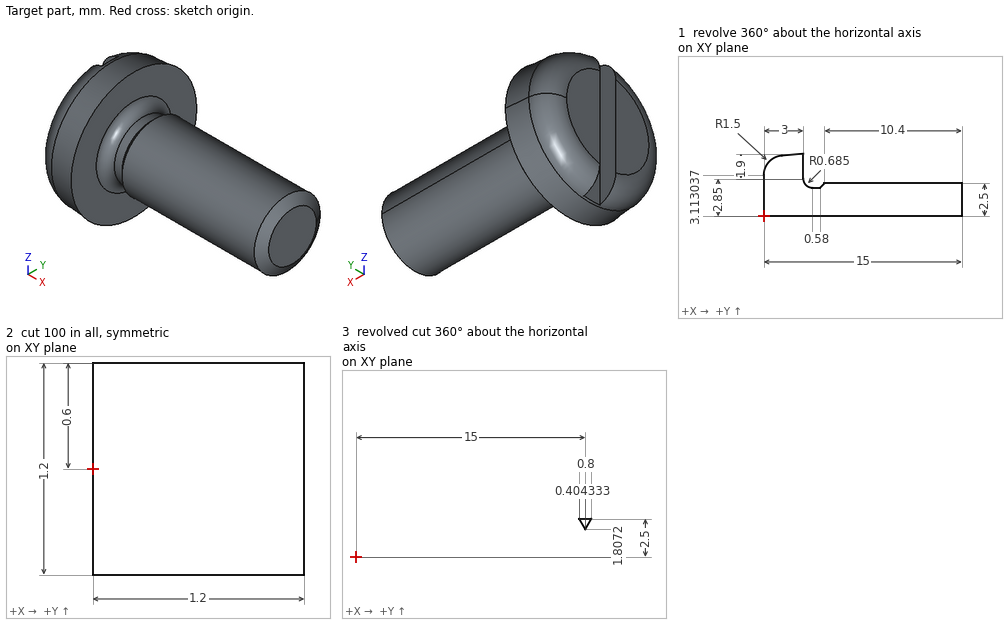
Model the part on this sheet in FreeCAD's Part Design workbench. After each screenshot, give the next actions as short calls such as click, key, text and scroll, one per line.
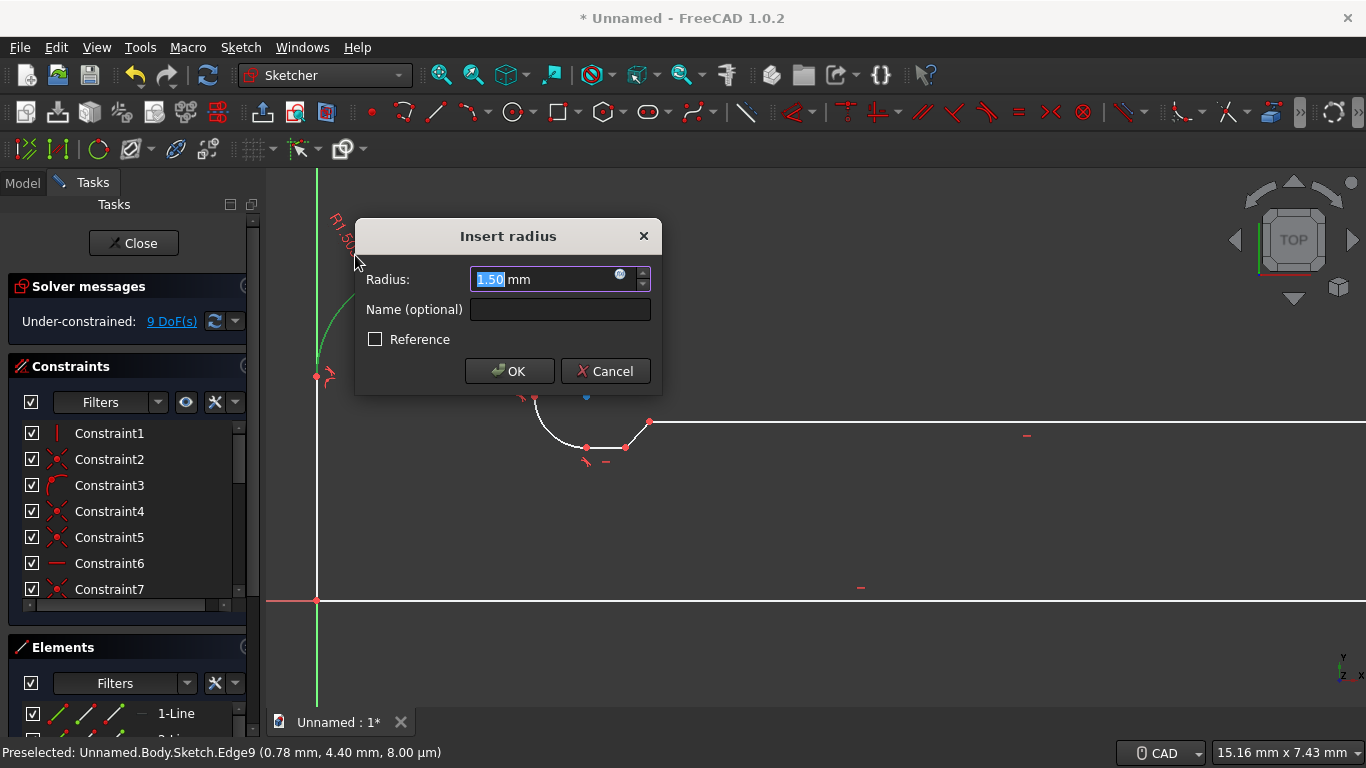
text(1.5)
key(Return)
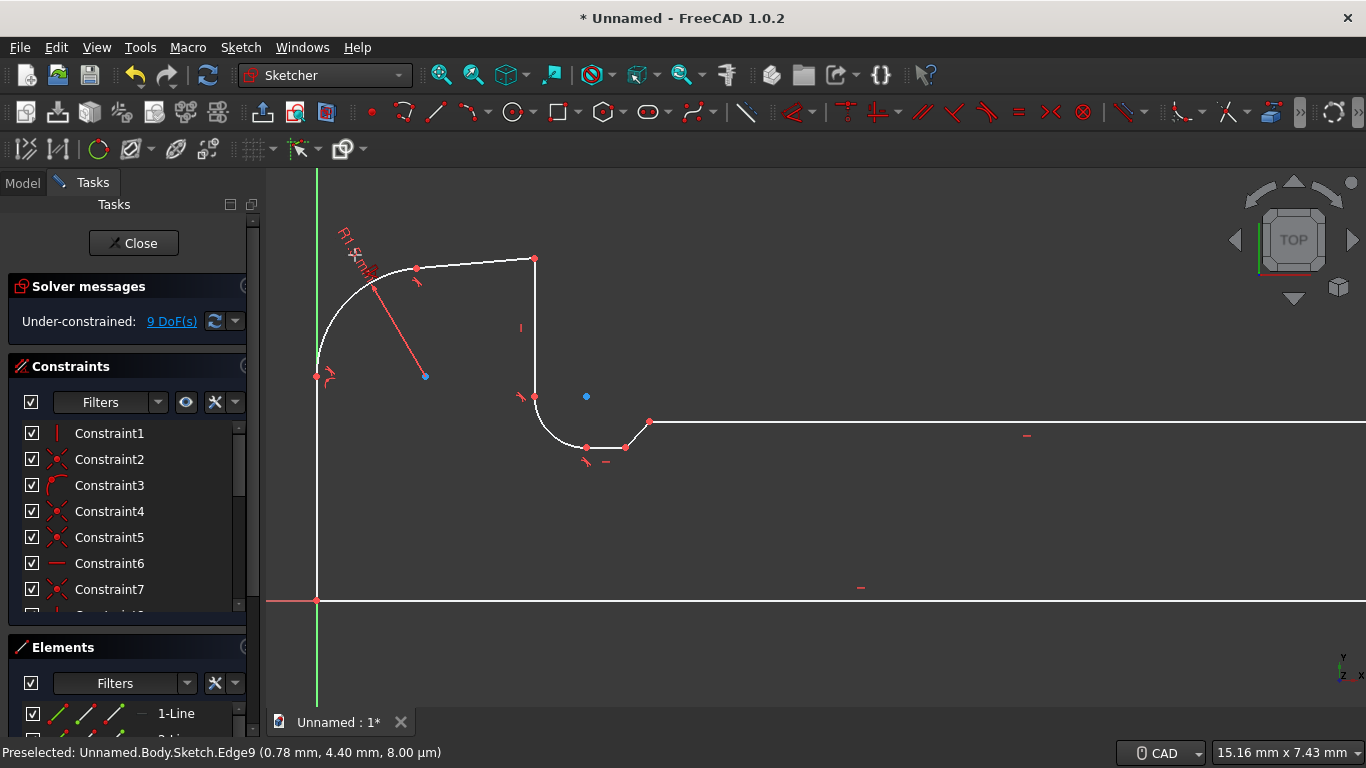
click(540, 420)
click(511, 435)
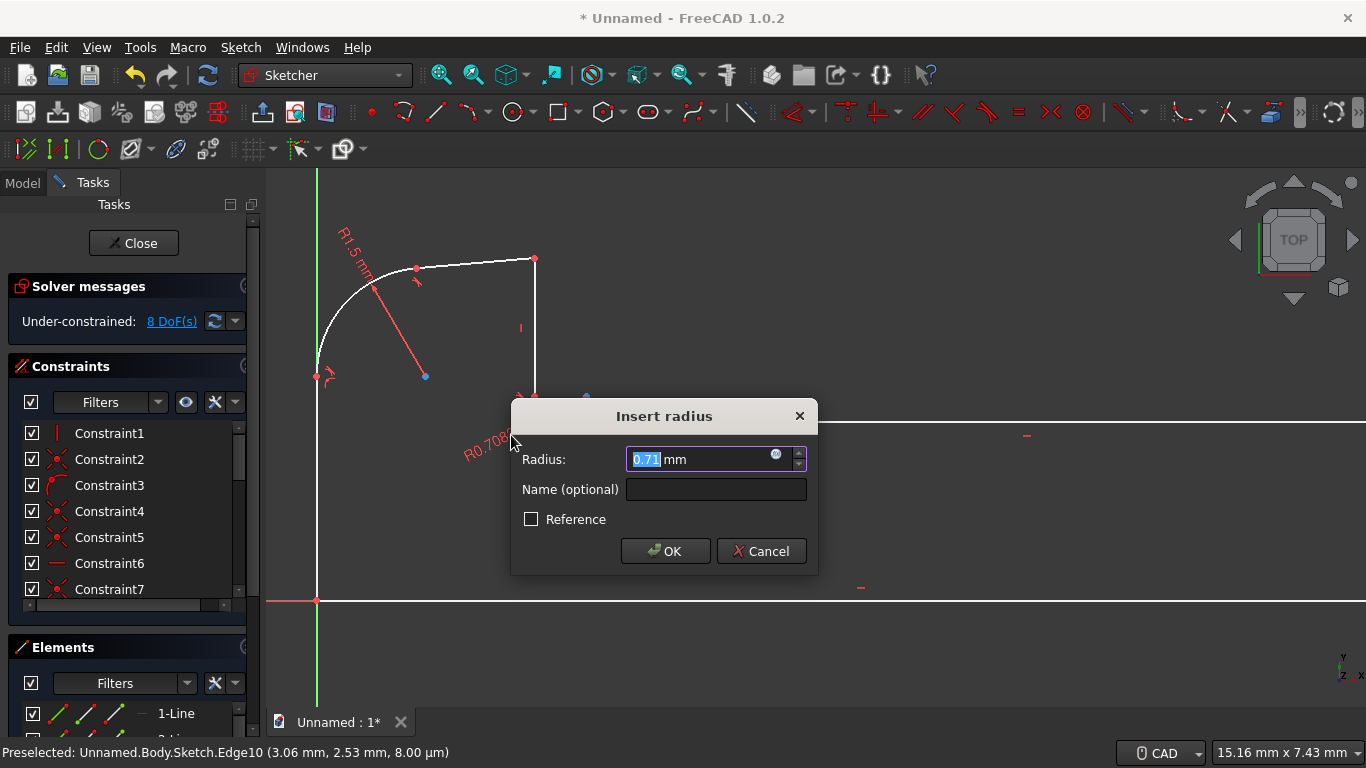
text(0.685)
key(Return)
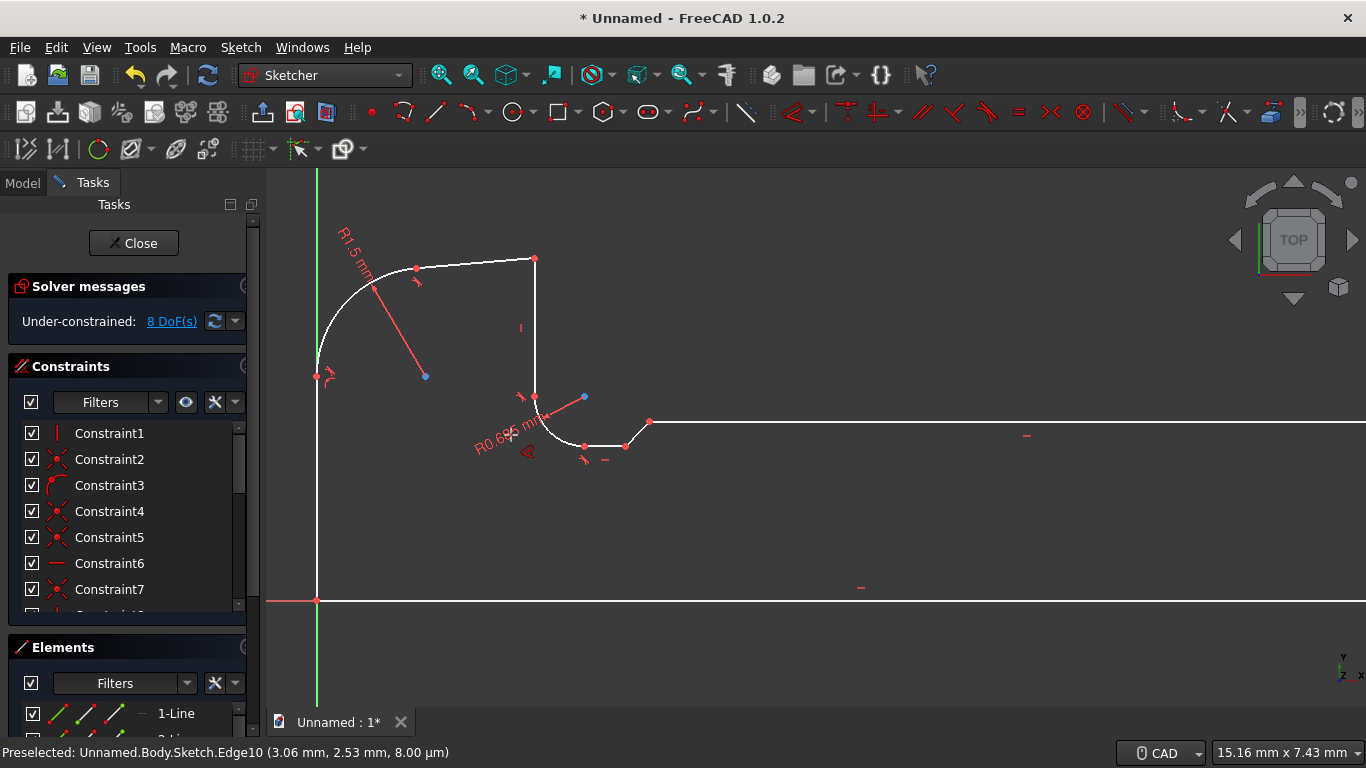
click(643, 601)
click(759, 635)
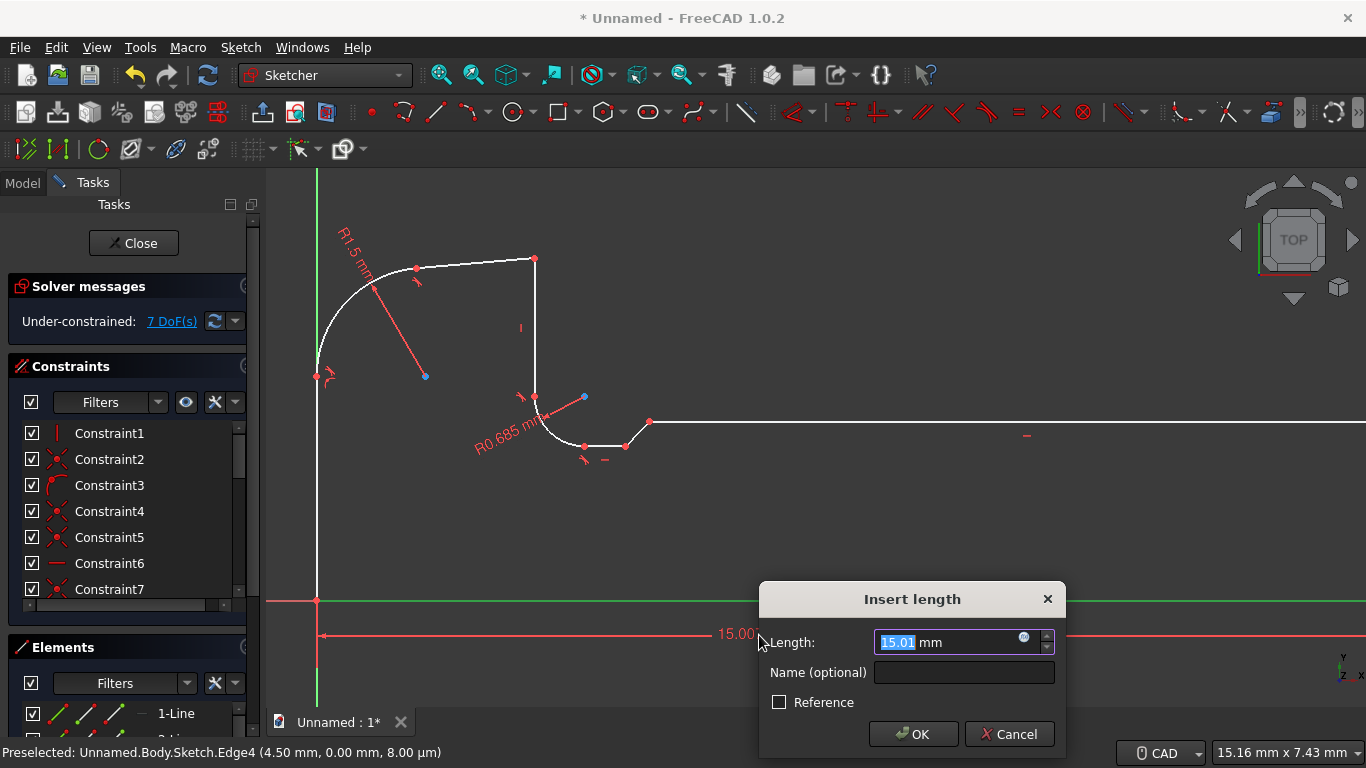
text(15)
key(Return)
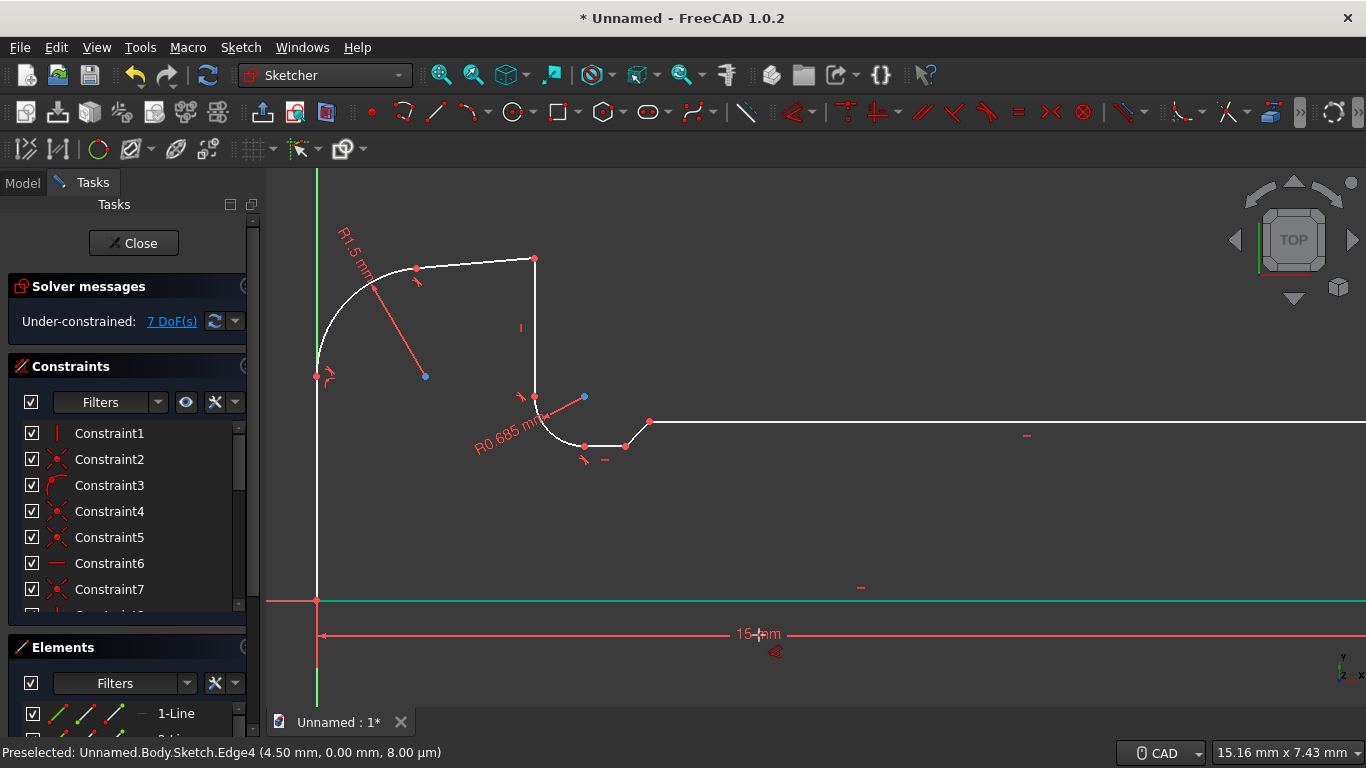
click(535, 396)
click(426, 635)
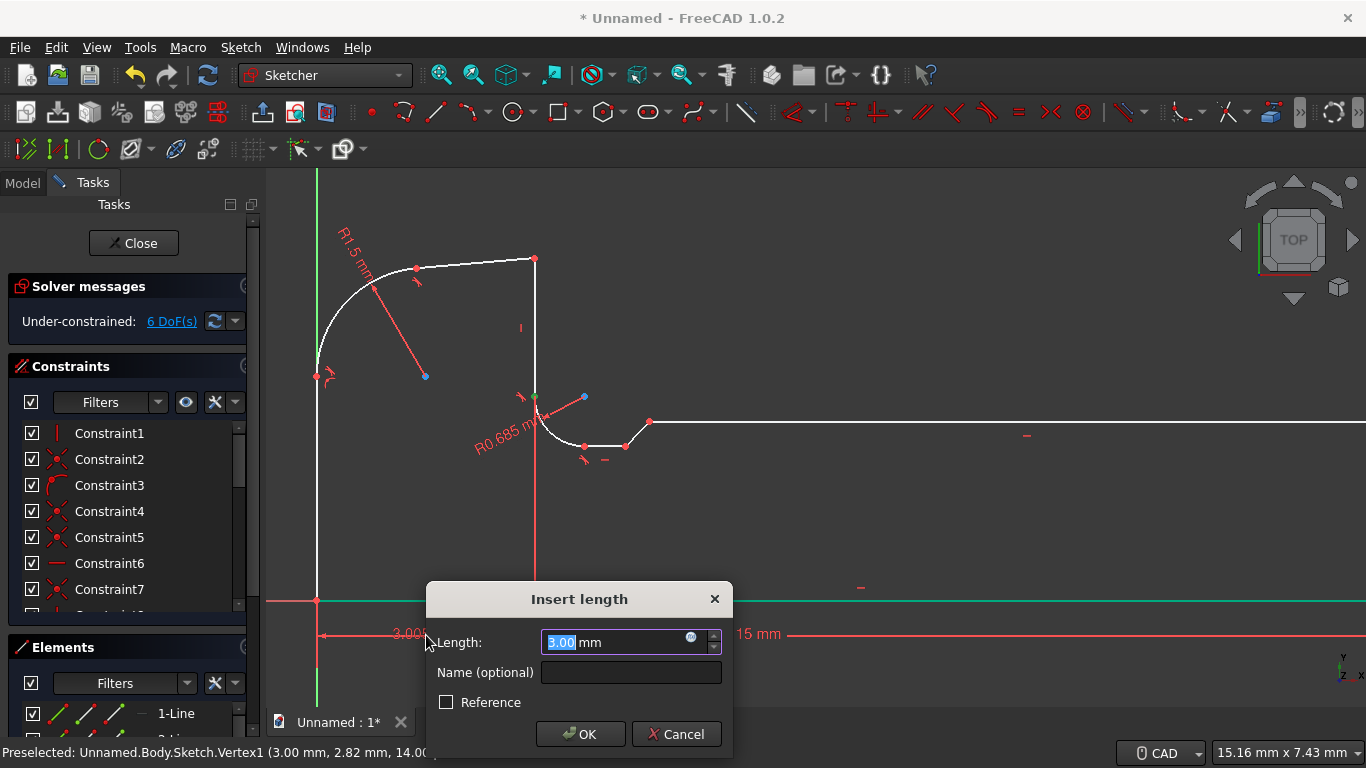
text(3)
key(Return)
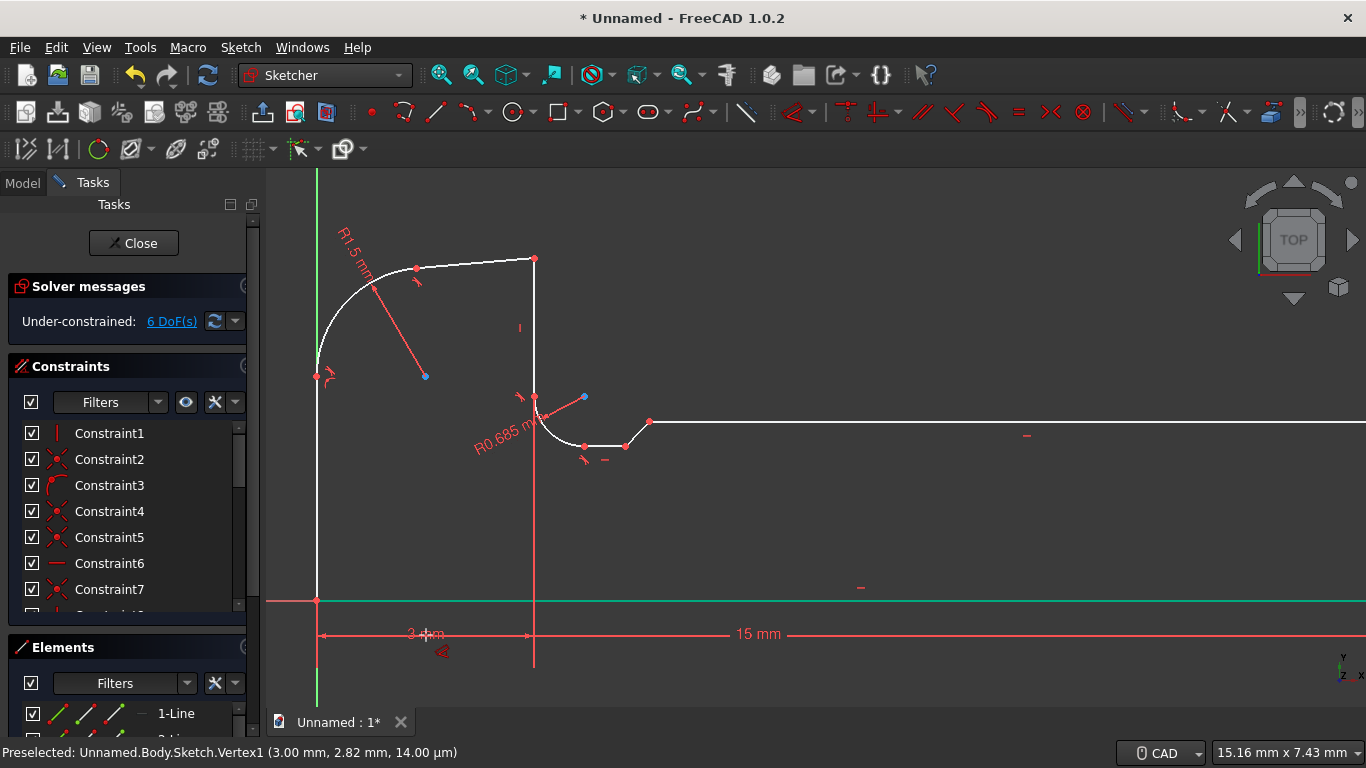
click(534, 355)
click(500, 327)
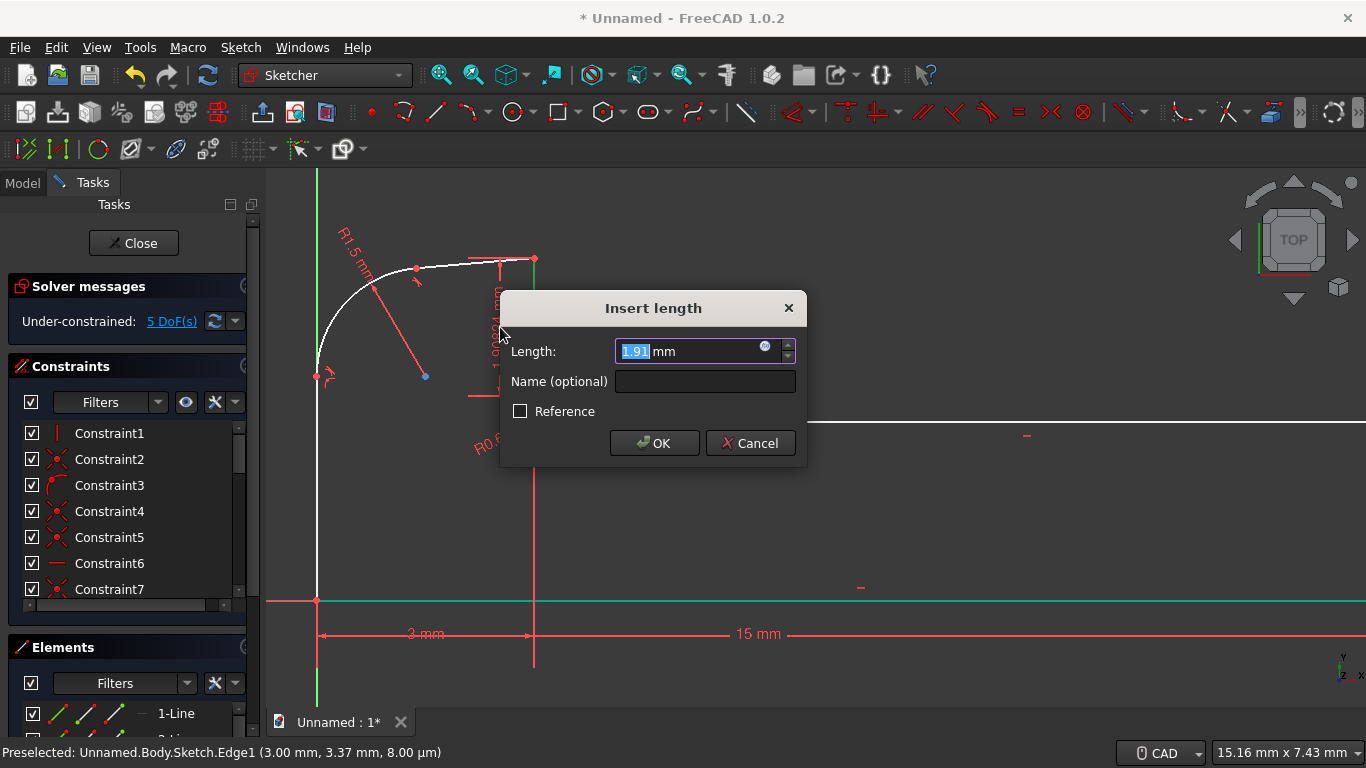
text(1.9)
key(Return)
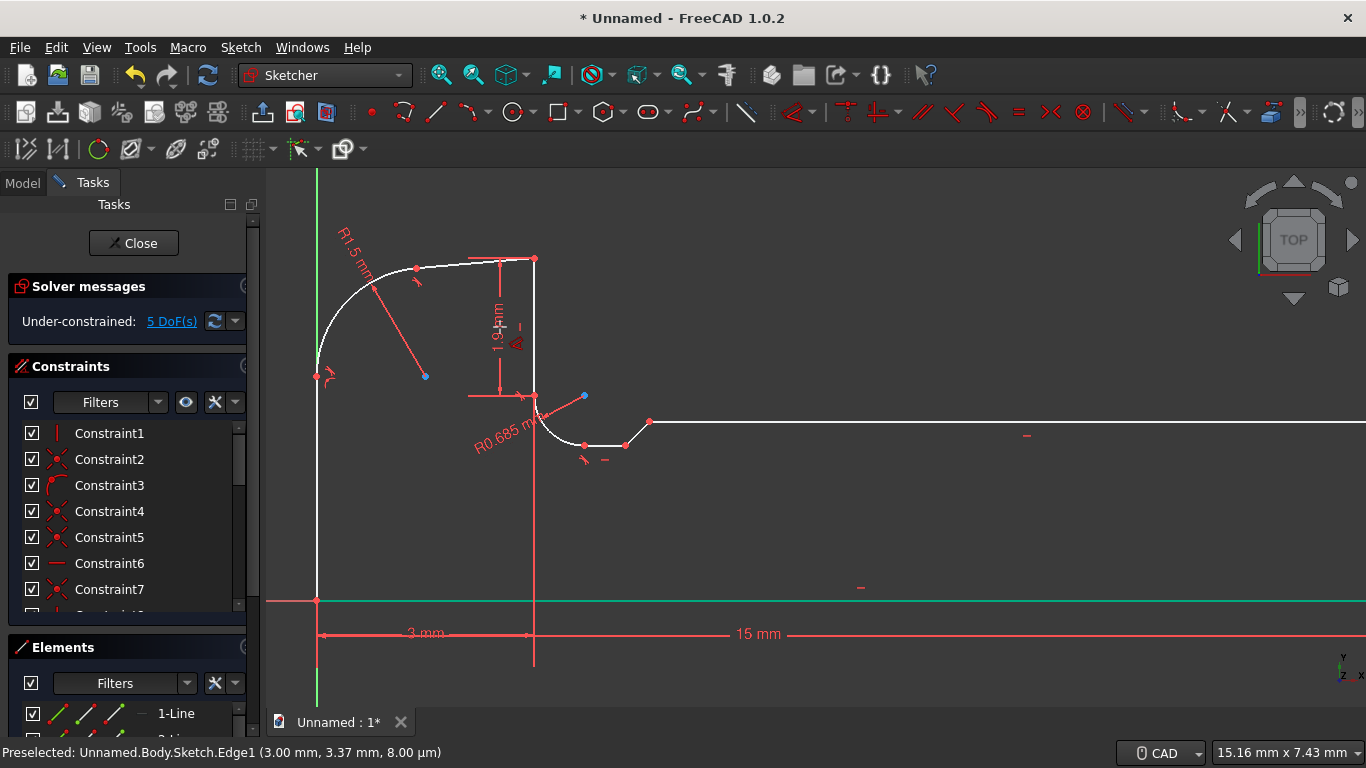
scroll(609, 449, down, 3)